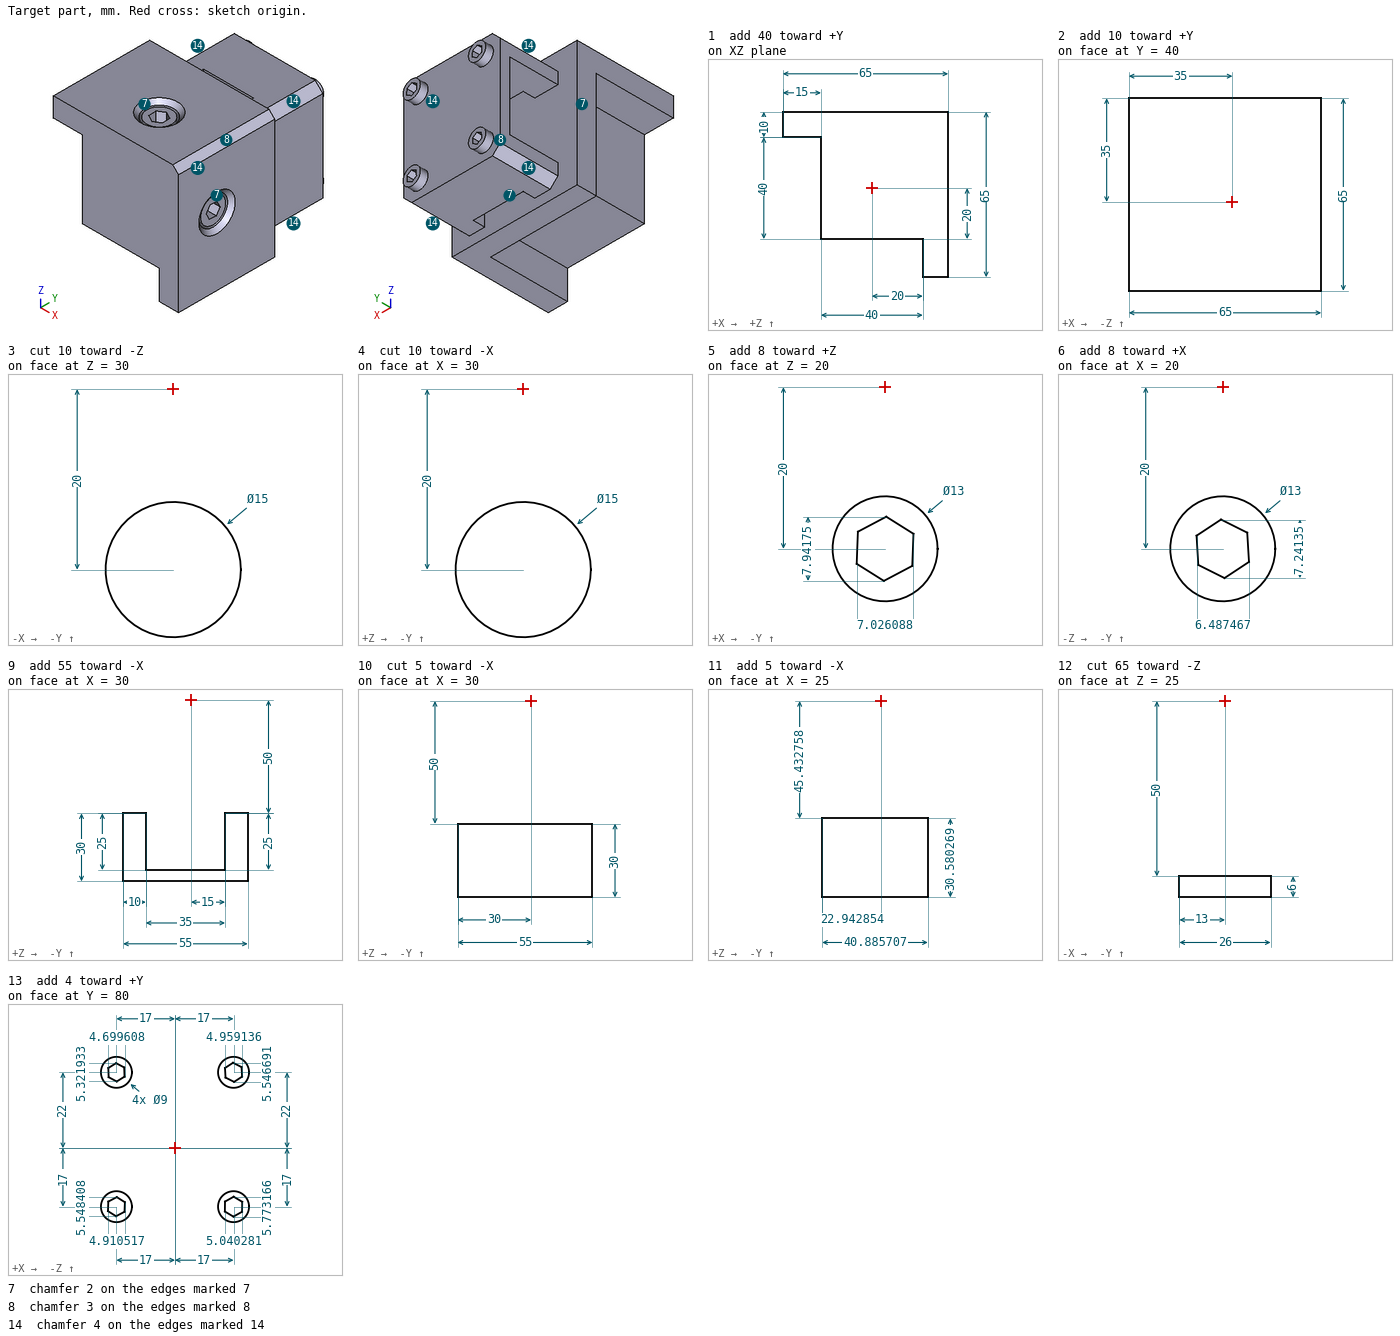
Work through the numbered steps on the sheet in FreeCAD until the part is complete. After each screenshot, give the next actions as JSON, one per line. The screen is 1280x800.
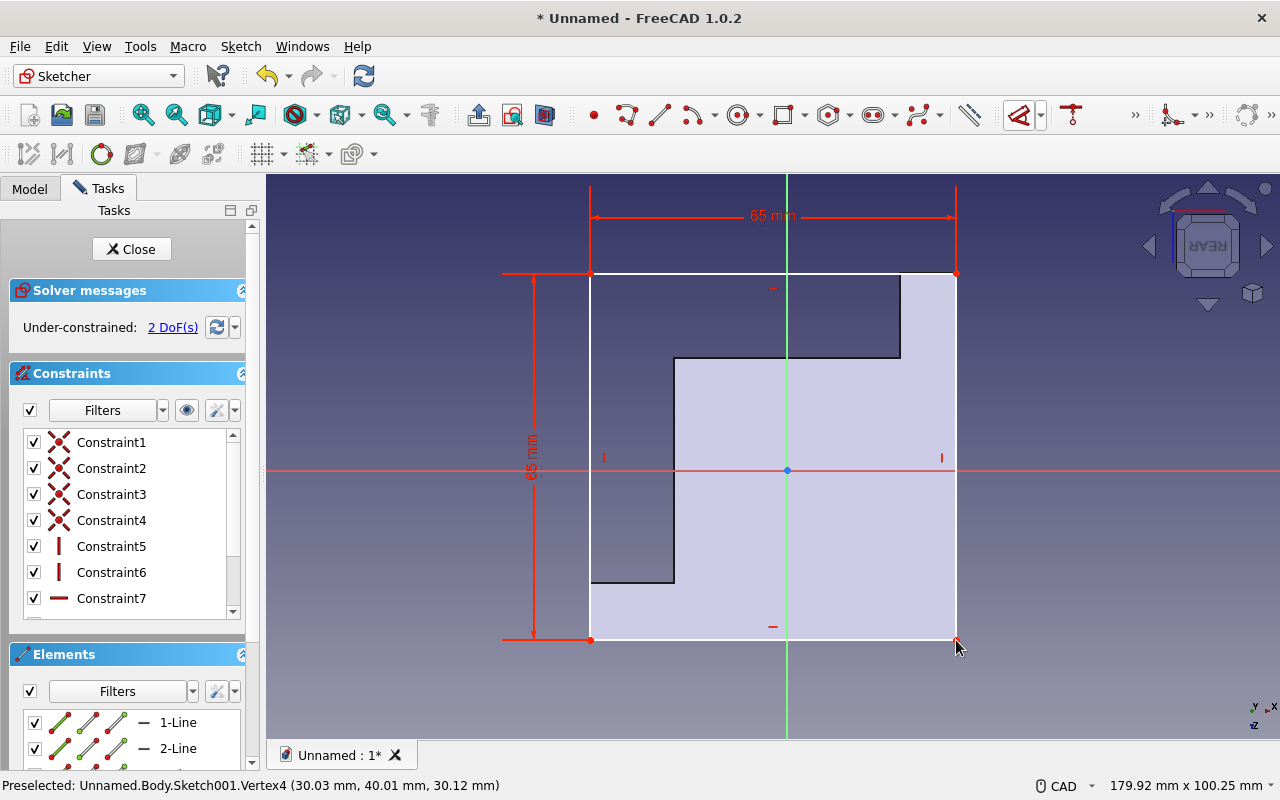
{"action": "left_click", "coordinate": [590, 274]}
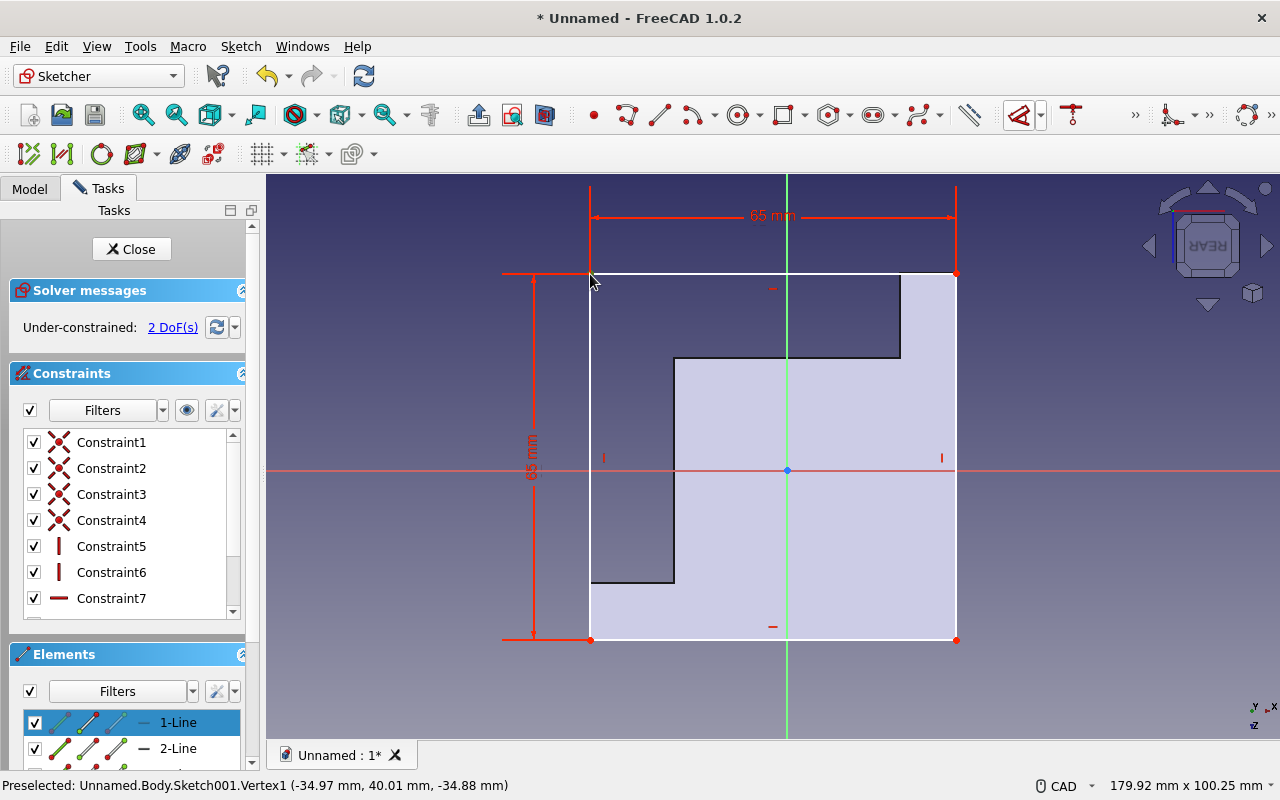
{"action": "key", "text": "l"}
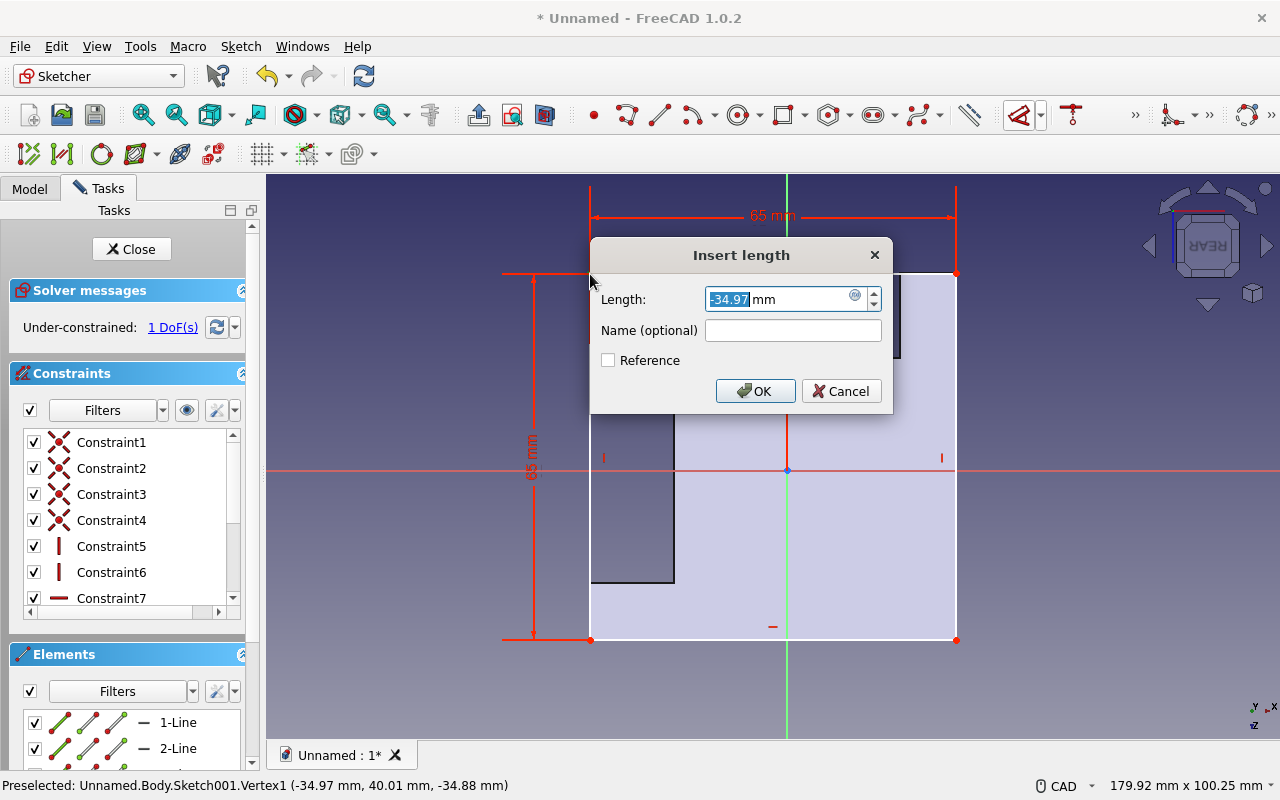
{"action": "type", "text": "-35"}
{"action": "key", "text": "Return"}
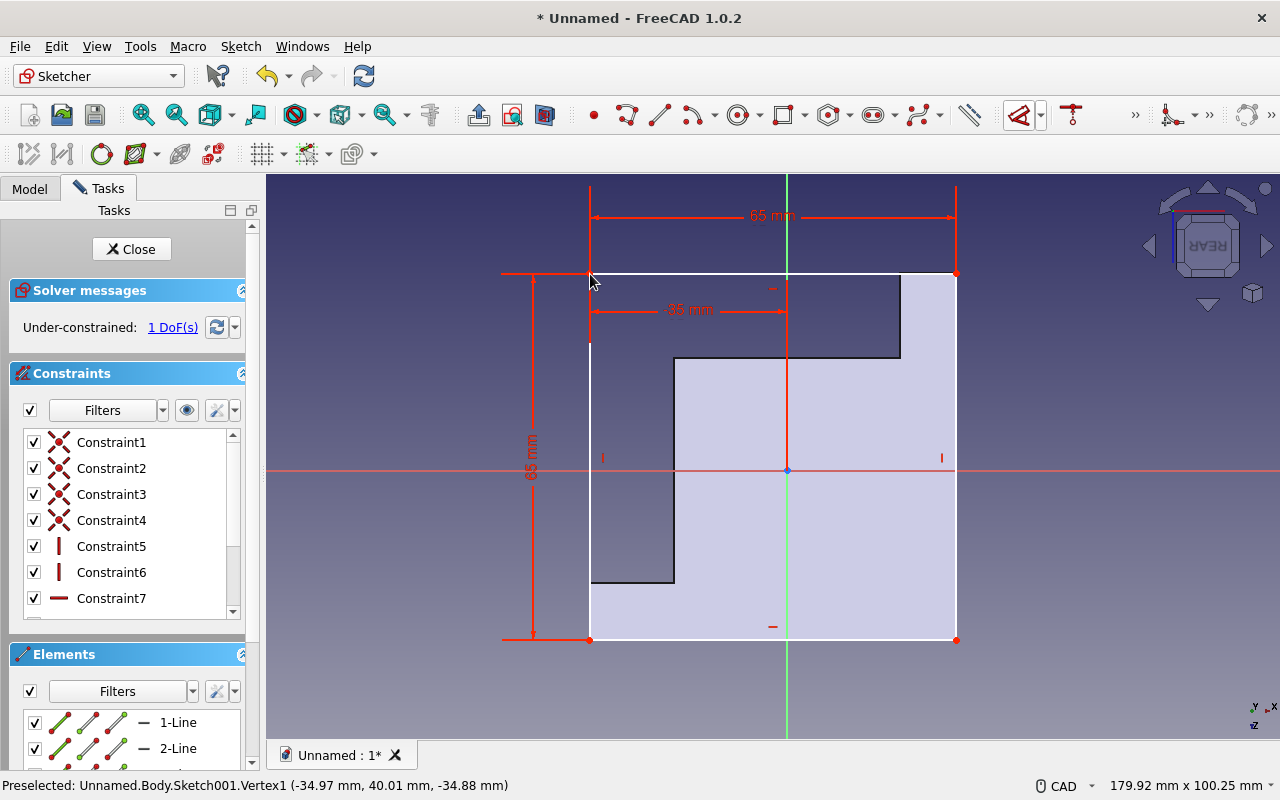
{"action": "left_click", "coordinate": [590, 274]}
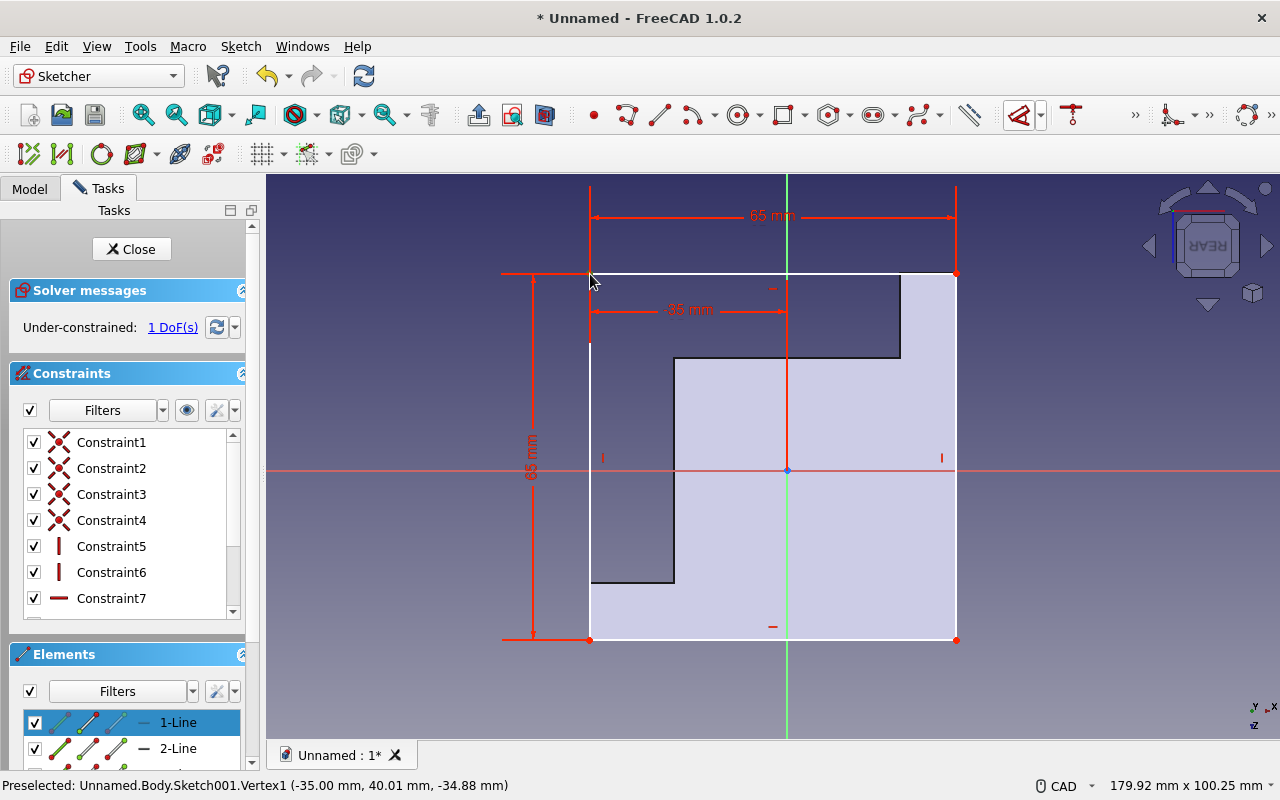
{"action": "left_click", "coordinate": [1040, 116]}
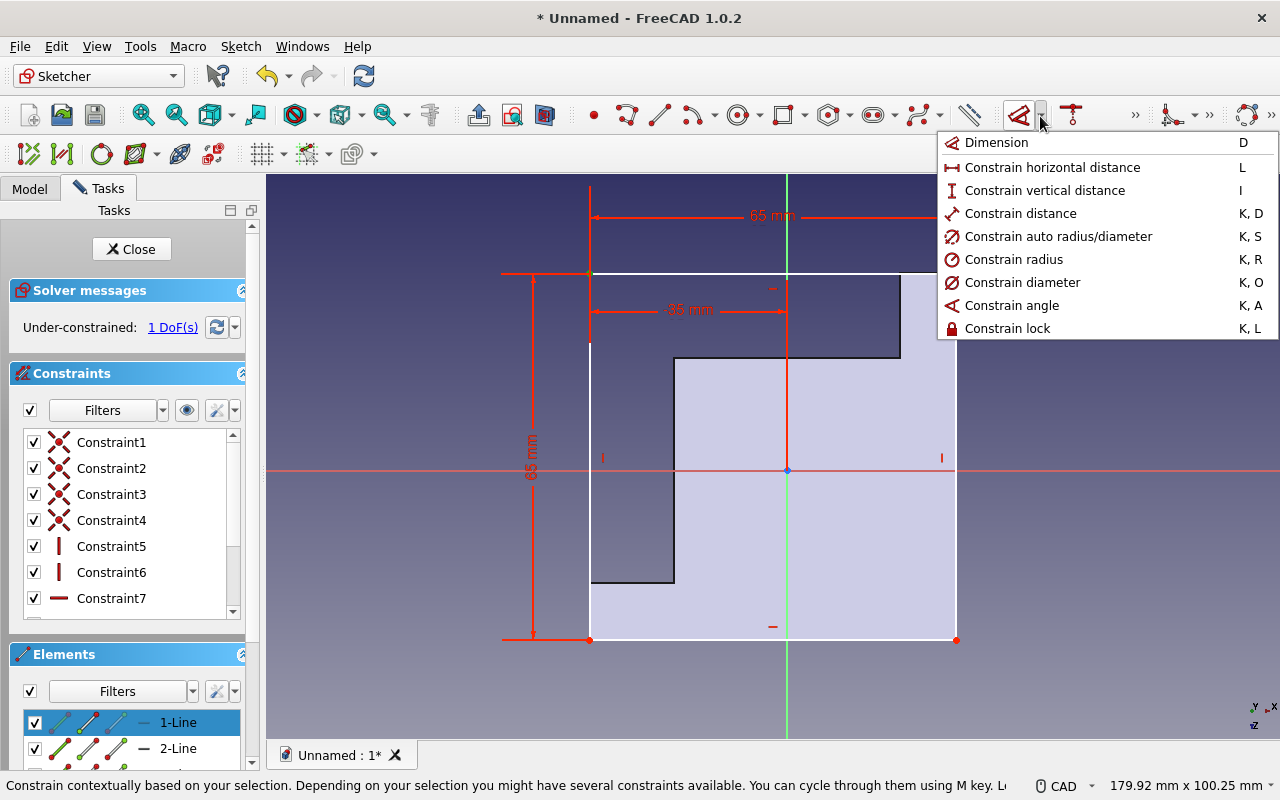
{"action": "left_click", "coordinate": [1108, 190]}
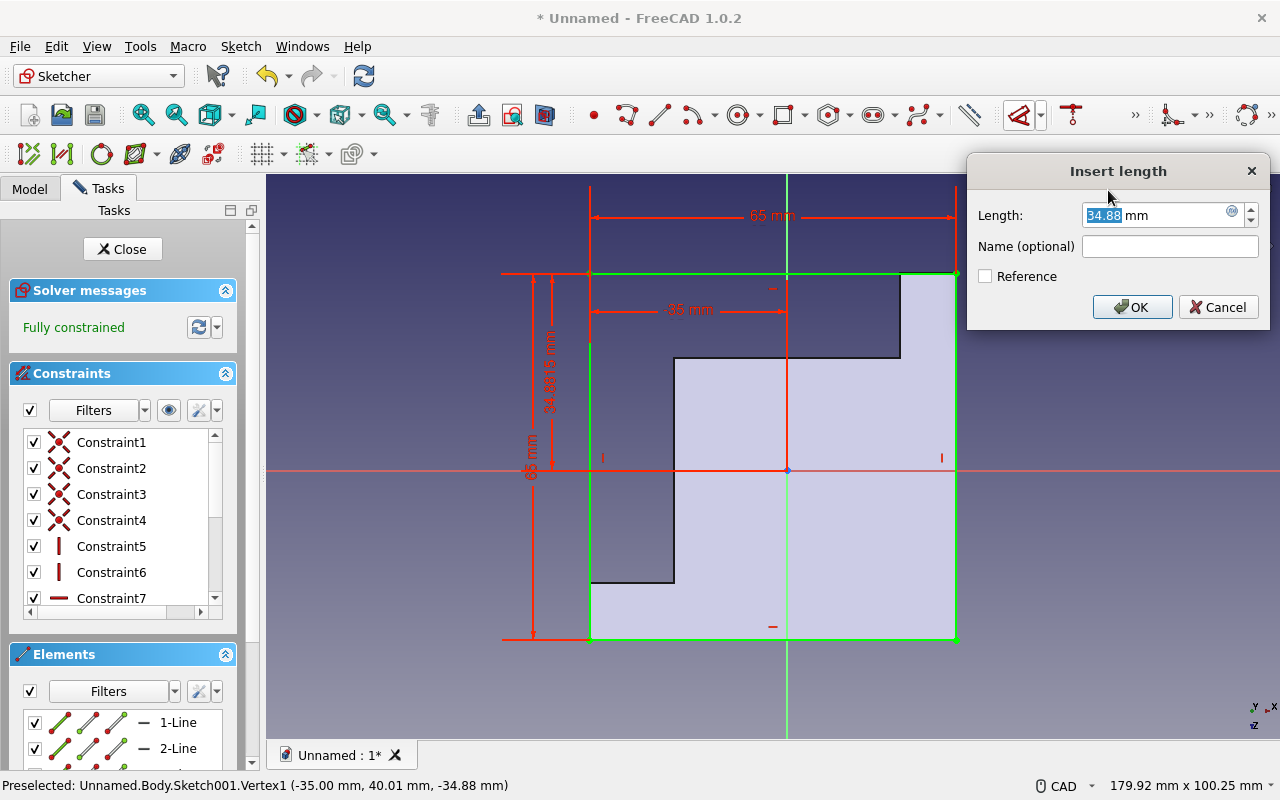
{"action": "type", "text": "35"}
{"action": "key", "text": "Return"}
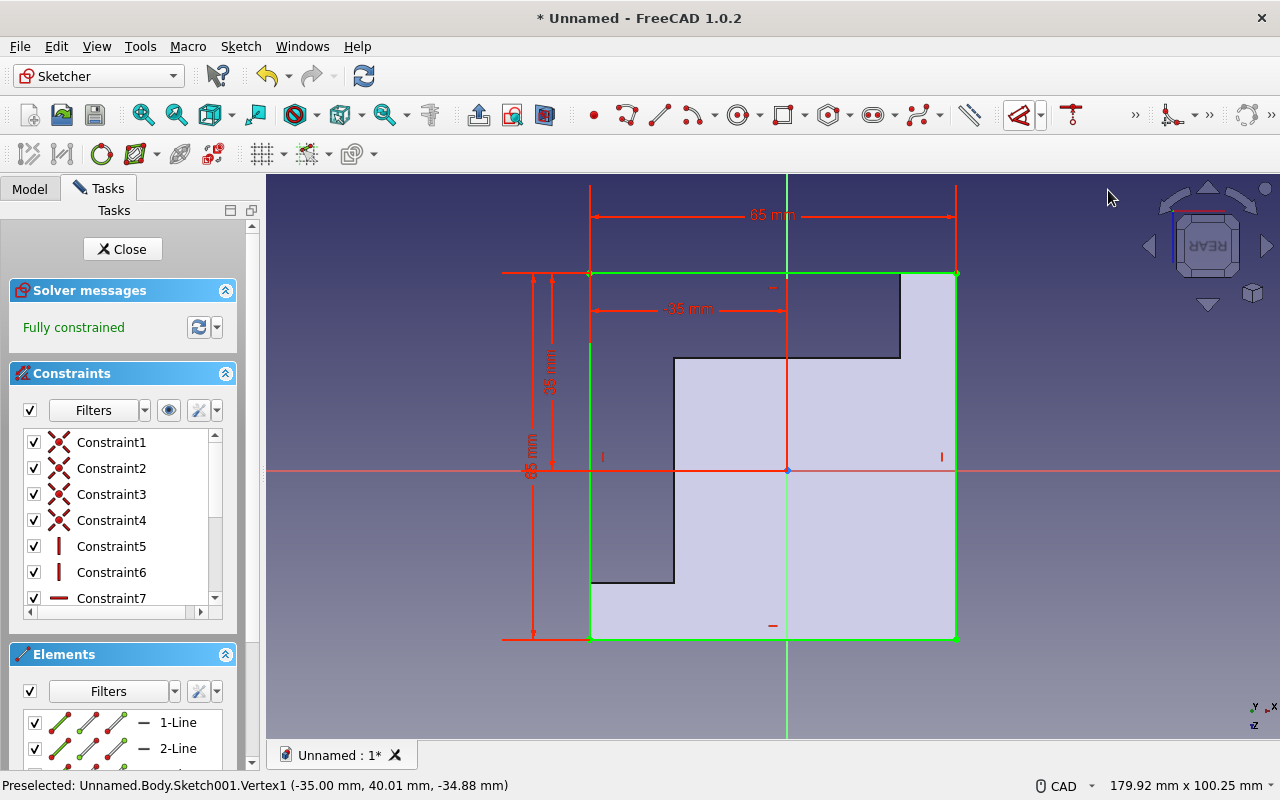
{"action": "left_click", "coordinate": [123, 249]}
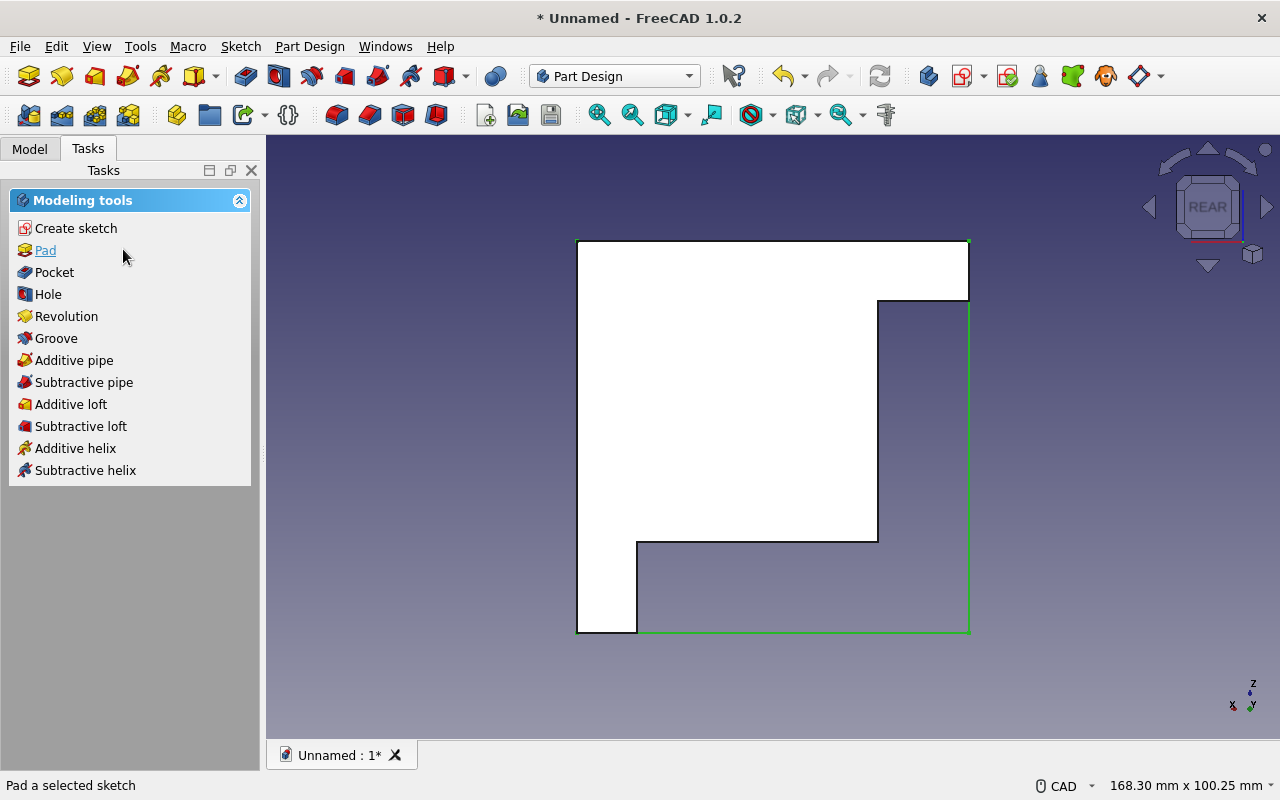
{"action": "left_click", "coordinate": [29, 76]}